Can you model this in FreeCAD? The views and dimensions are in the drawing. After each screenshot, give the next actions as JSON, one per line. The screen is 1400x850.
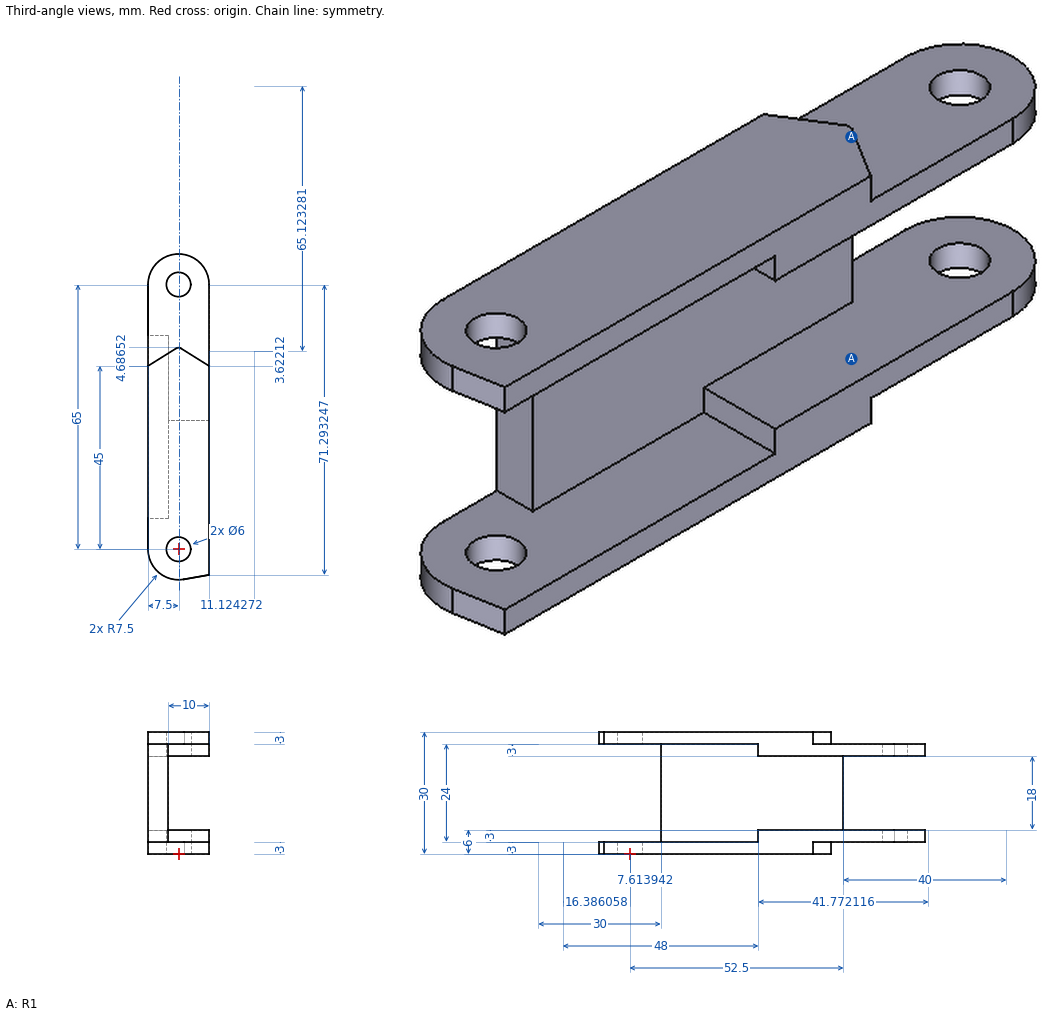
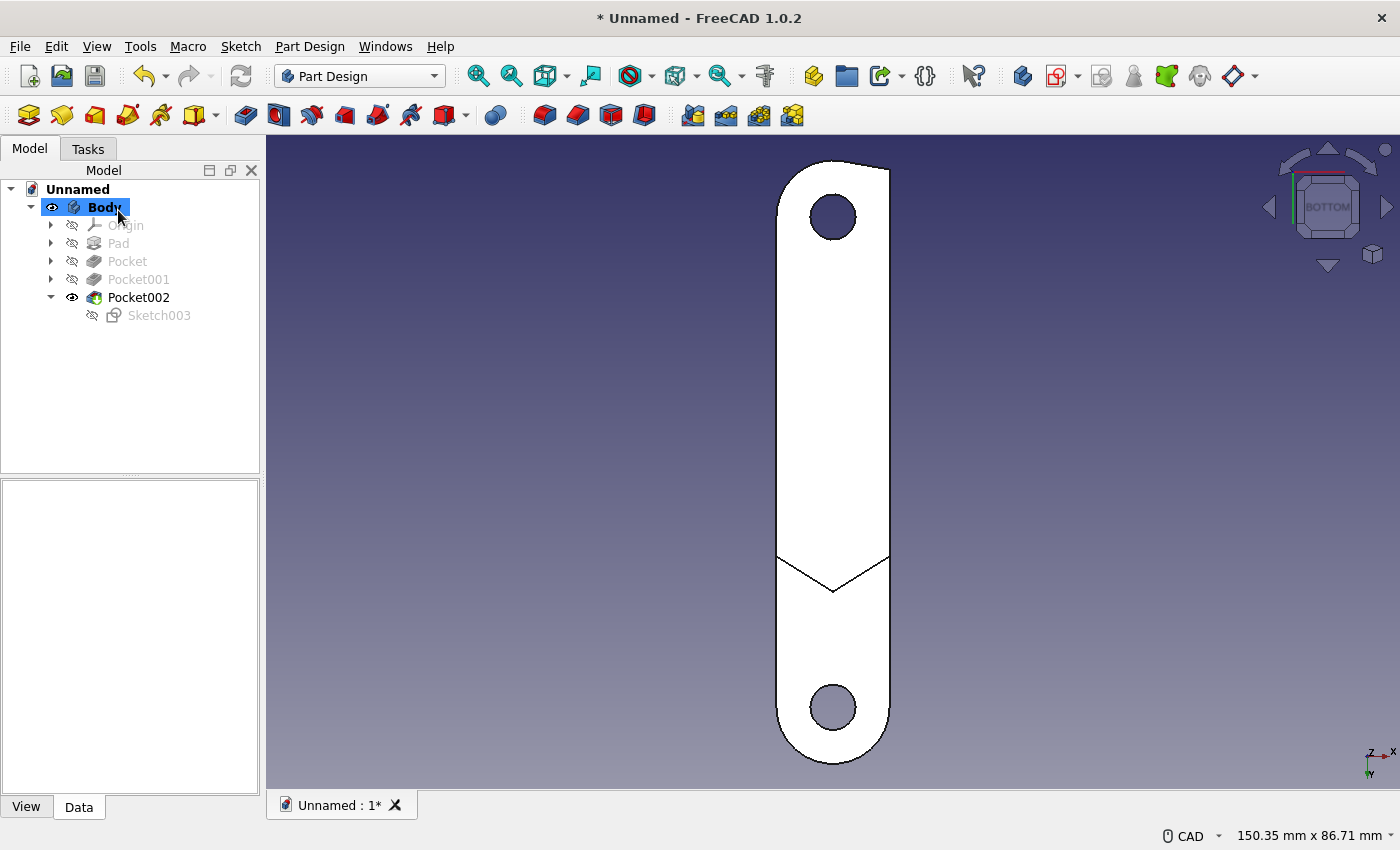
{"action": "key", "text": "0"}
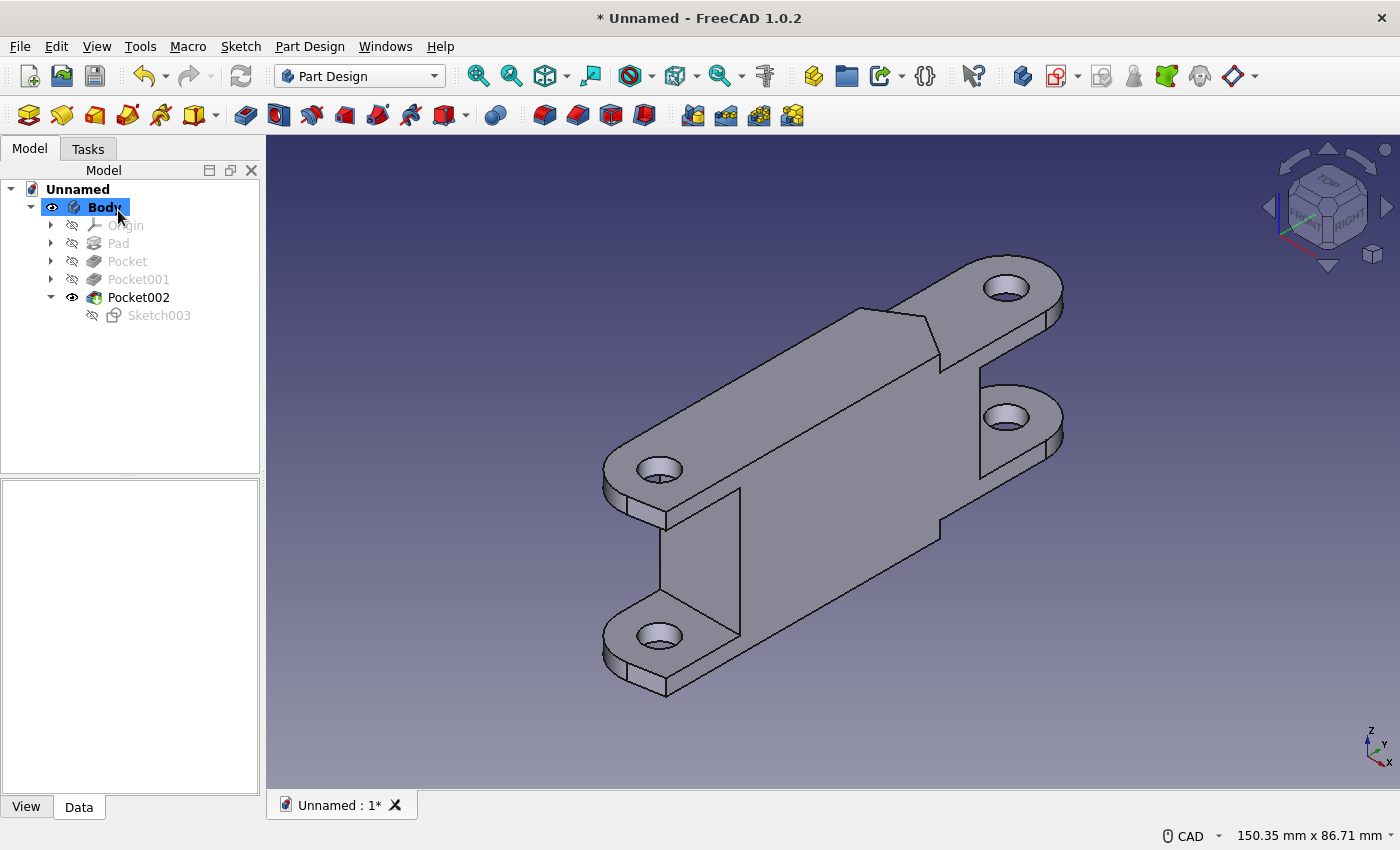
{"action": "key", "text": "2"}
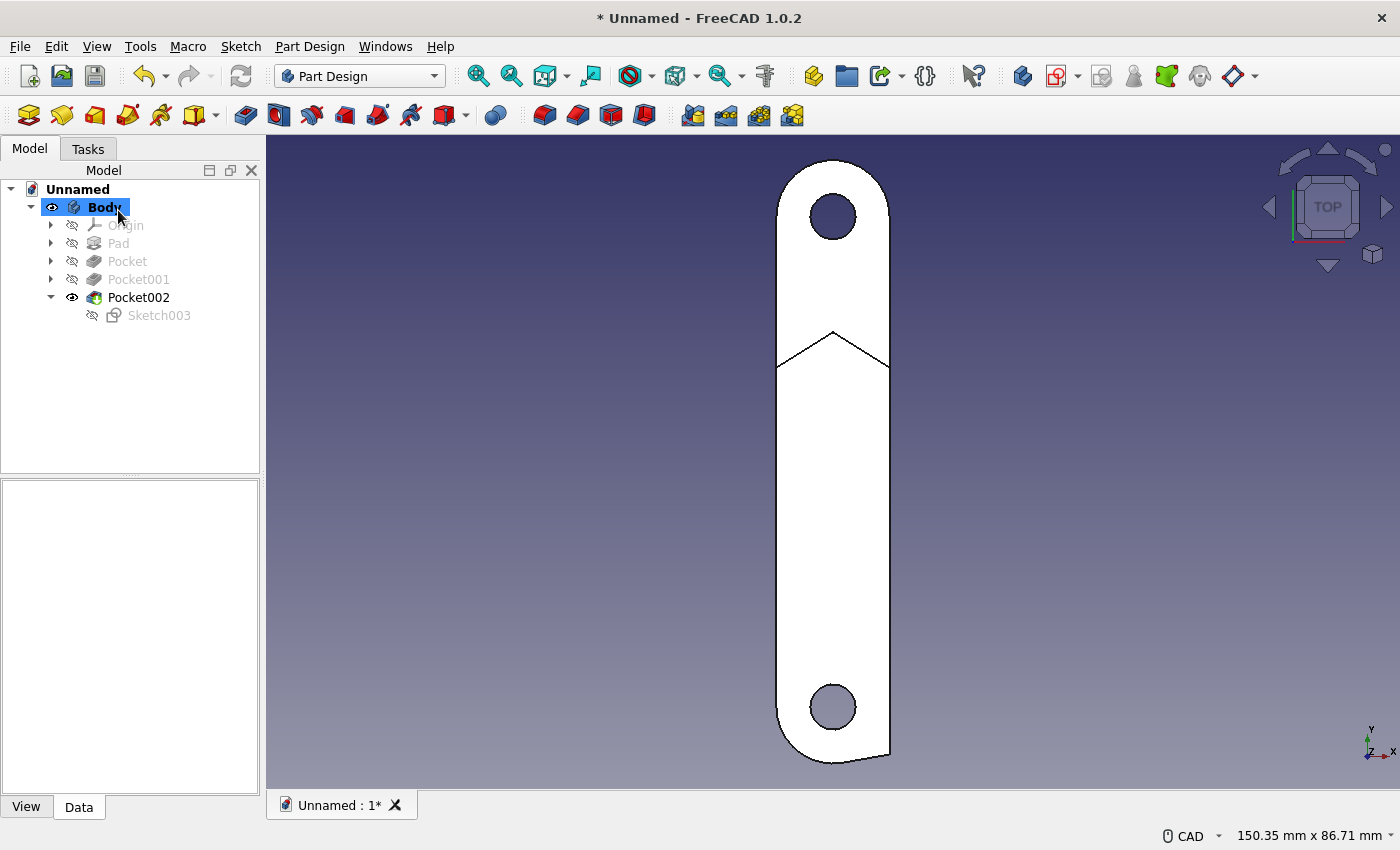
{"action": "key", "text": "1"}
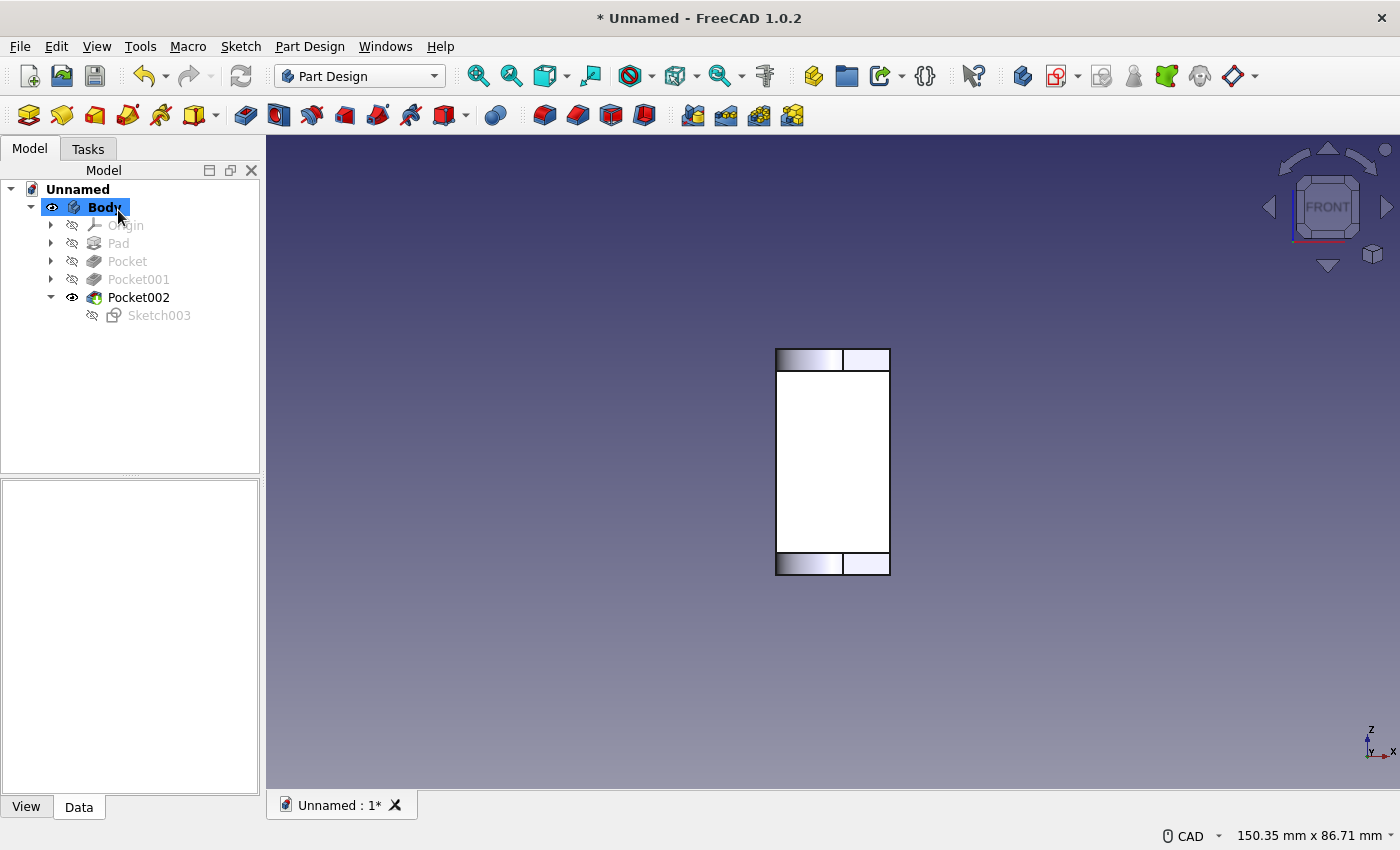
{"action": "key", "text": "v f"}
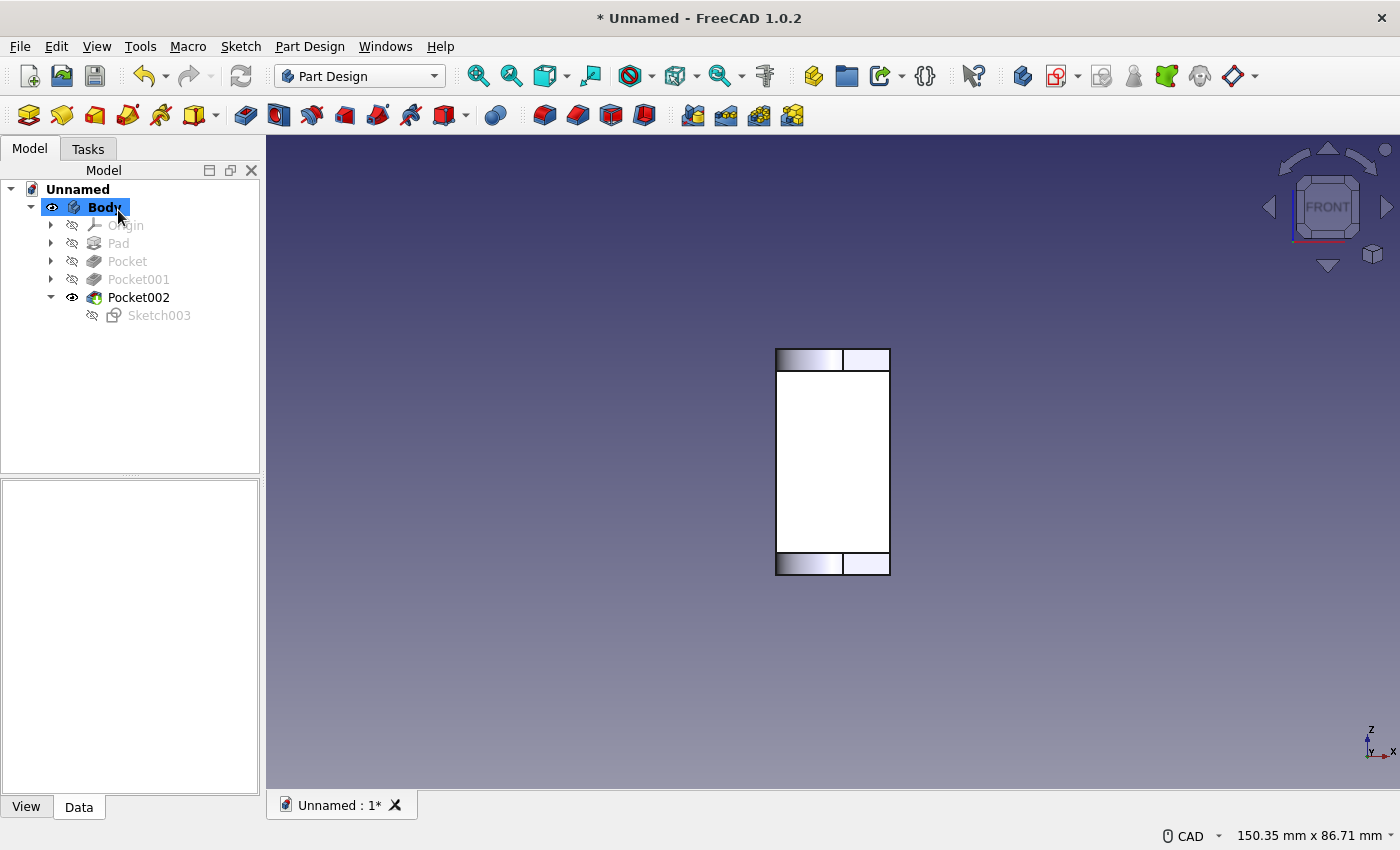
{"action": "key", "text": "3"}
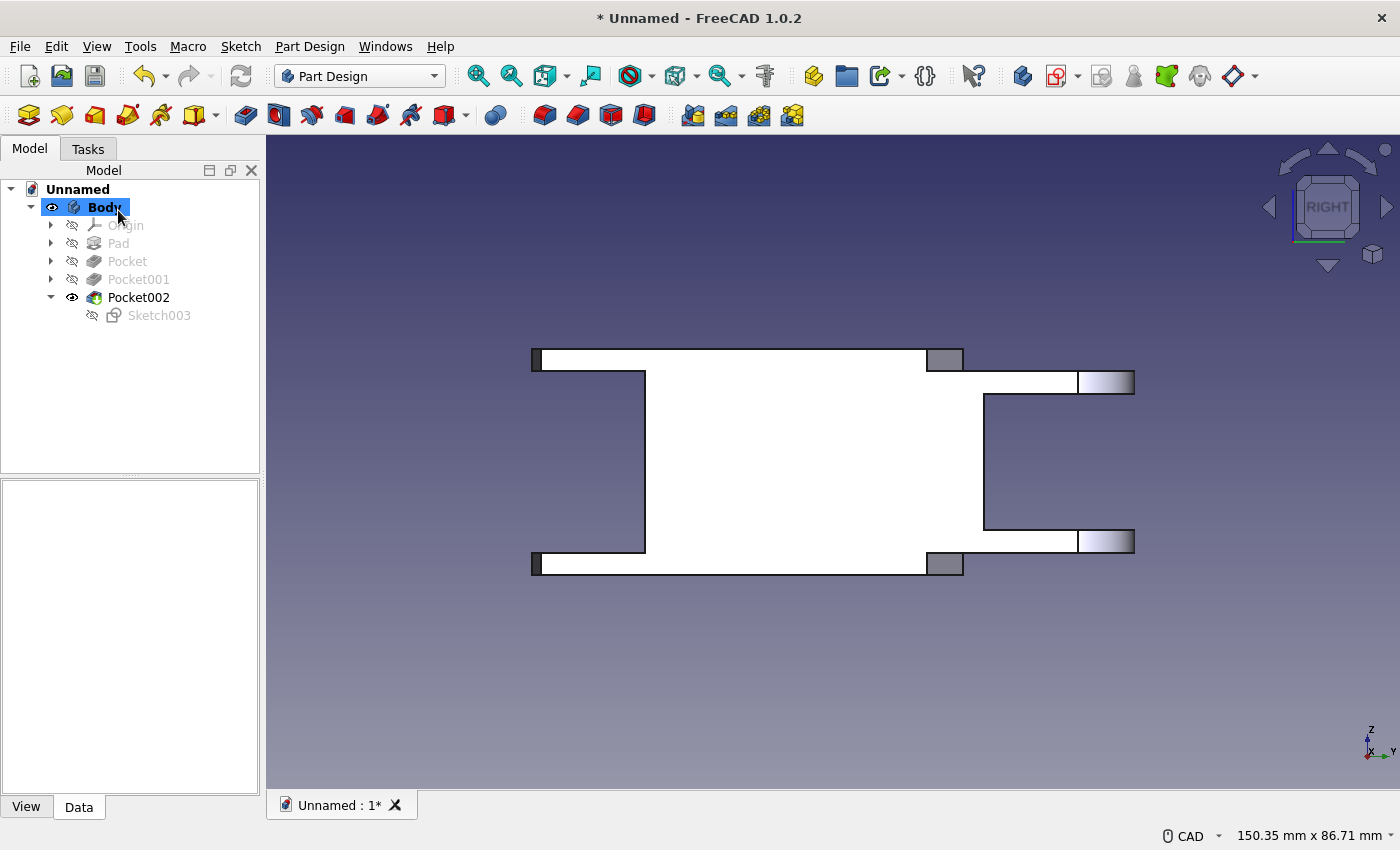
{"action": "key", "text": "5"}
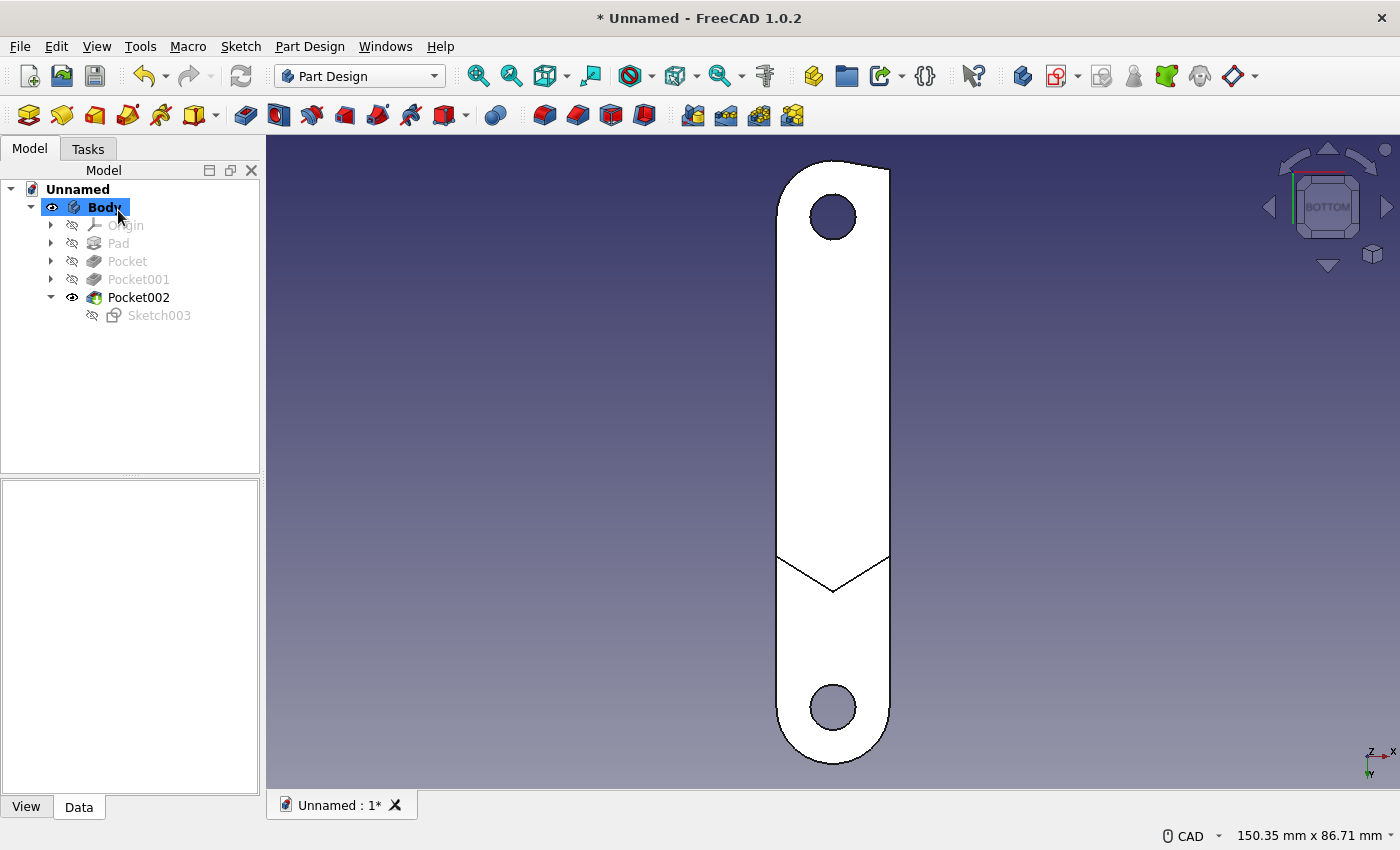
{"action": "key", "text": "4"}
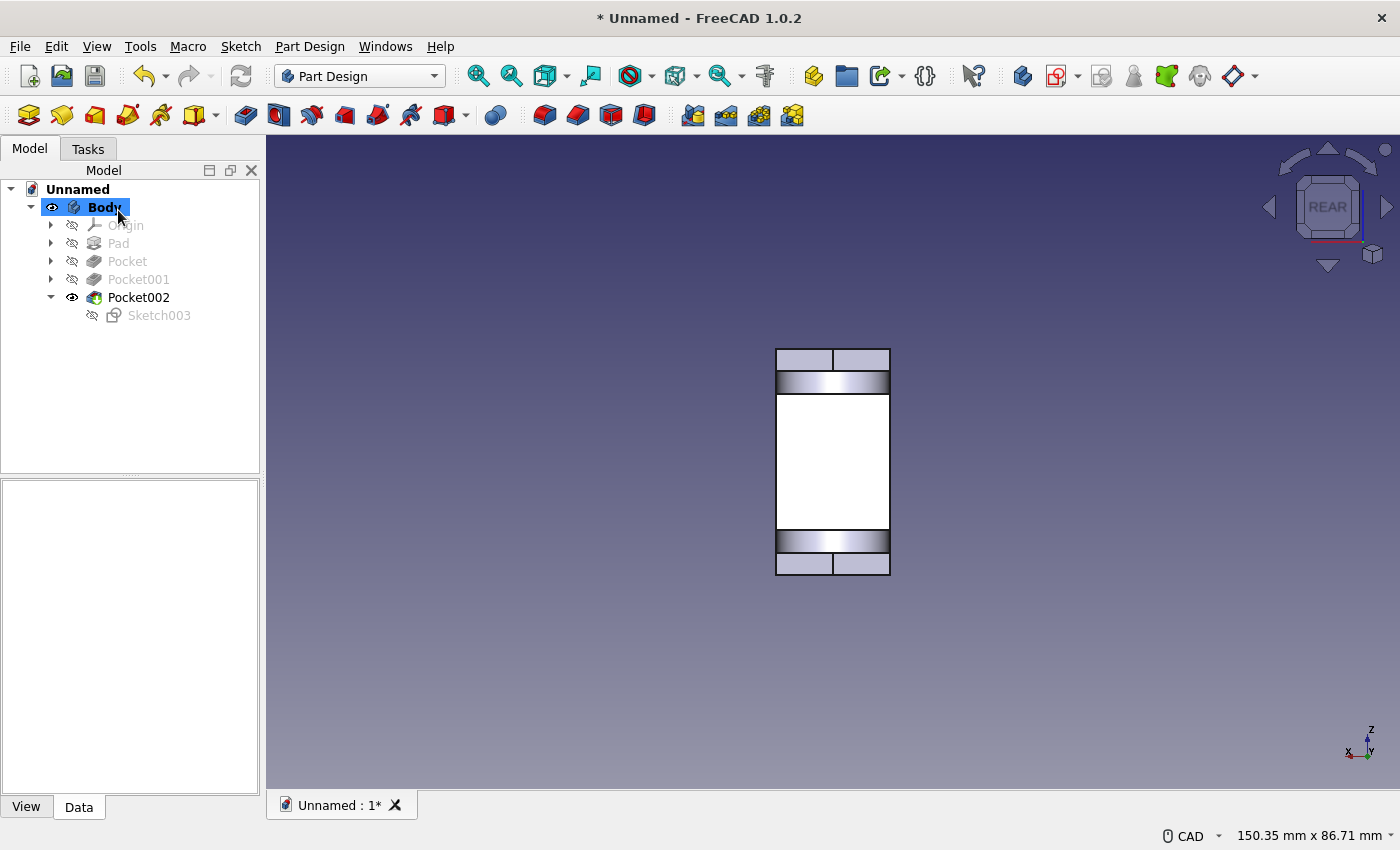
{"action": "key", "text": "v f"}